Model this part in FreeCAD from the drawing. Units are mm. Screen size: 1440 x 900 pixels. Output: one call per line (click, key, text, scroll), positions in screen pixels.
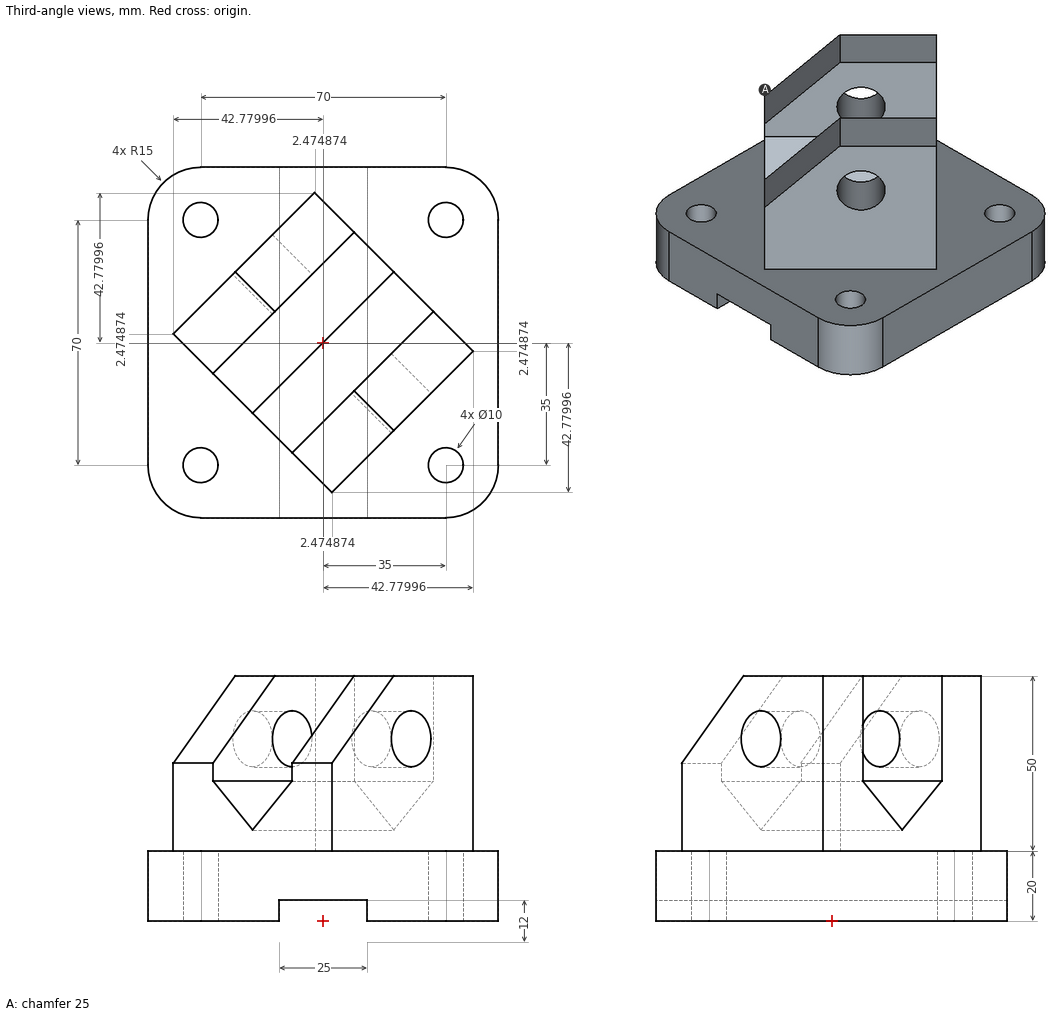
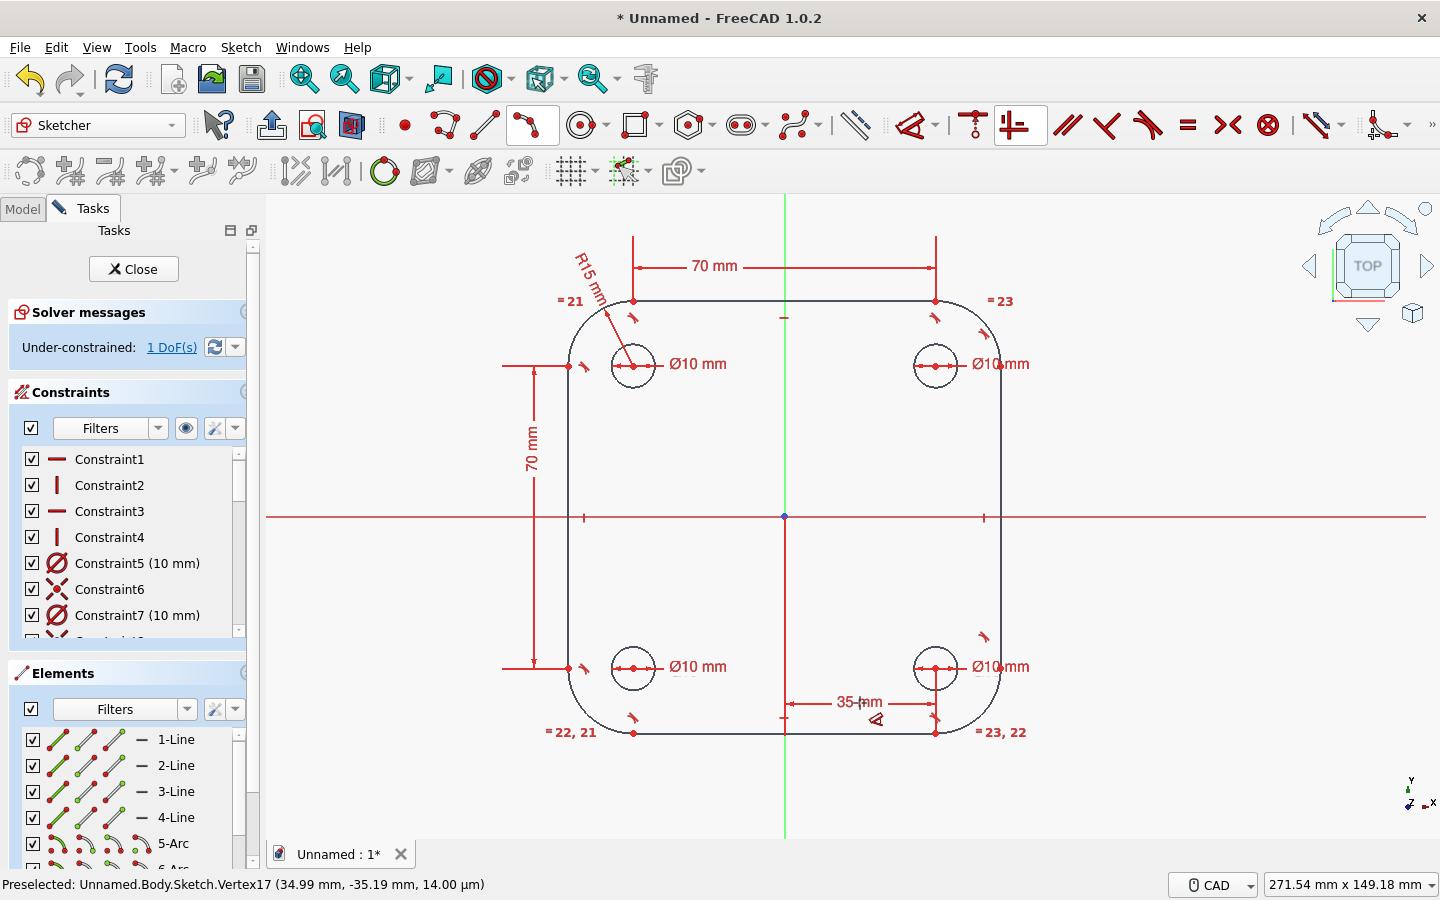
click(936, 669)
click(970, 593)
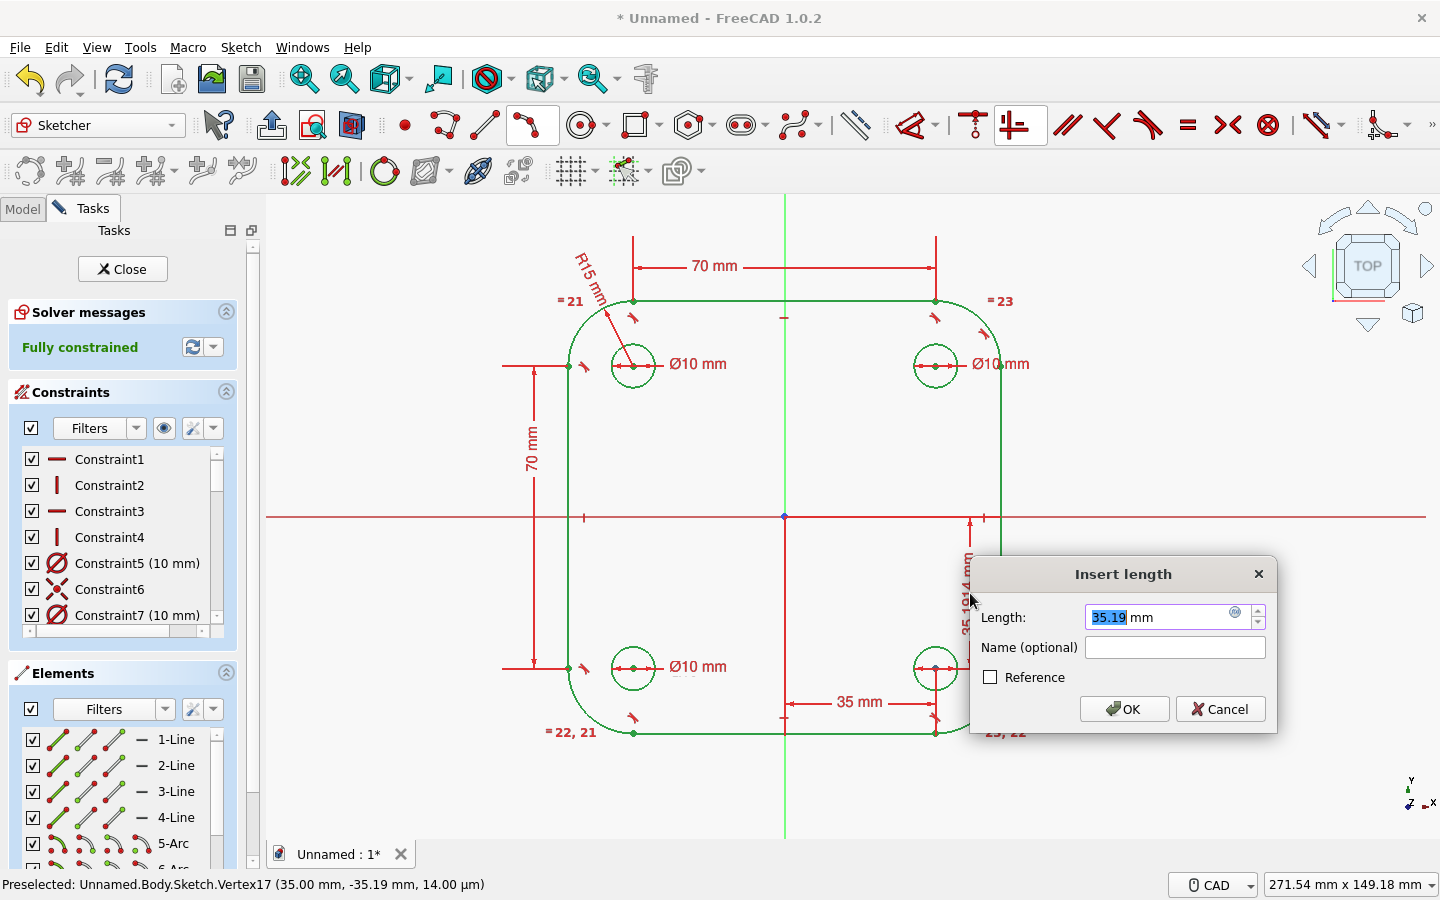
text(35)
key(Return)
key(Escape)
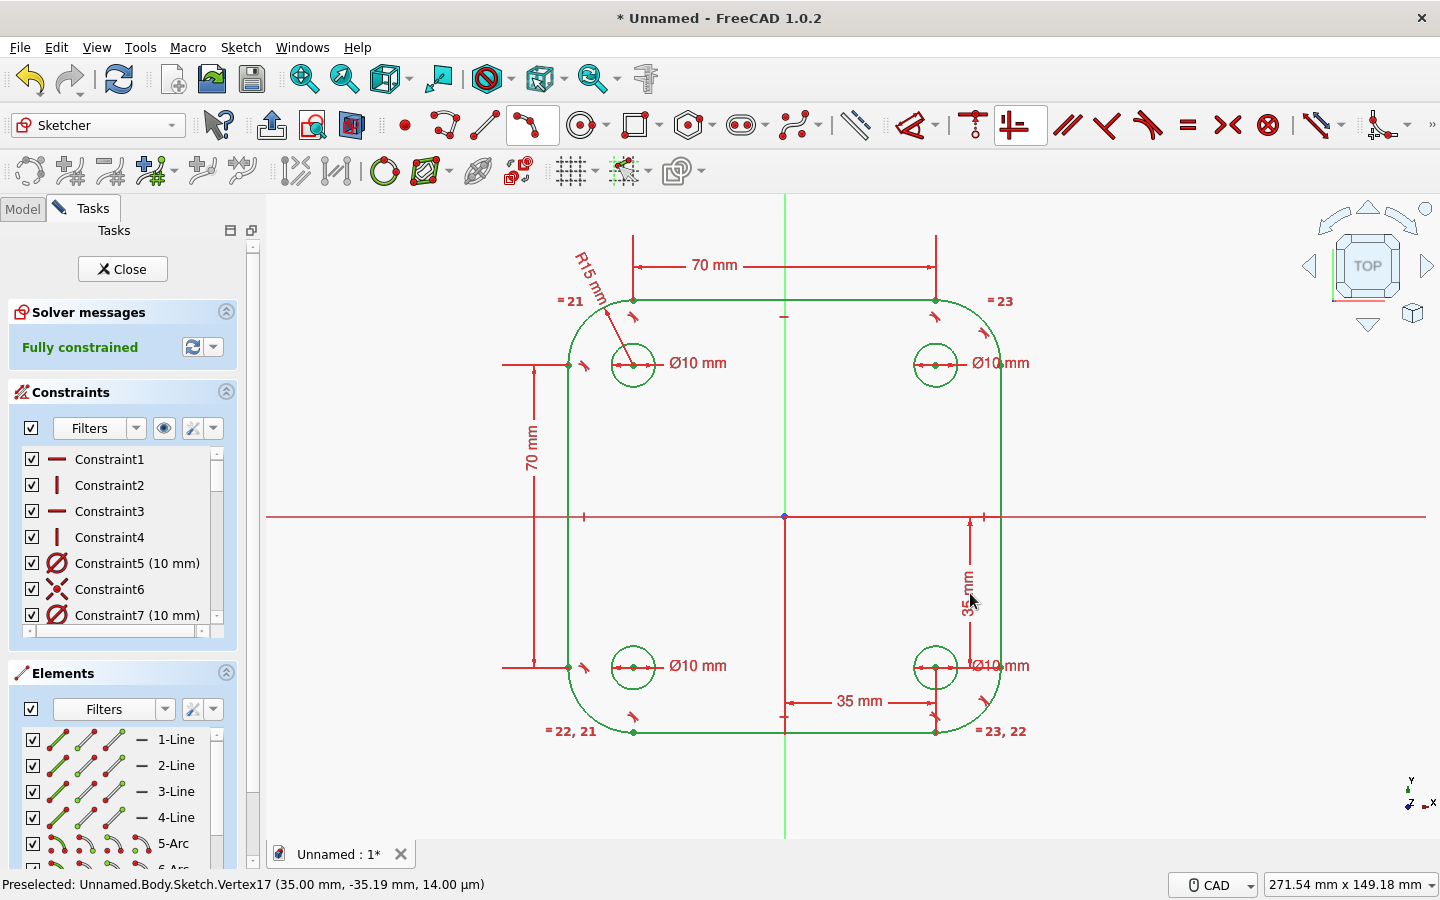
click(123, 269)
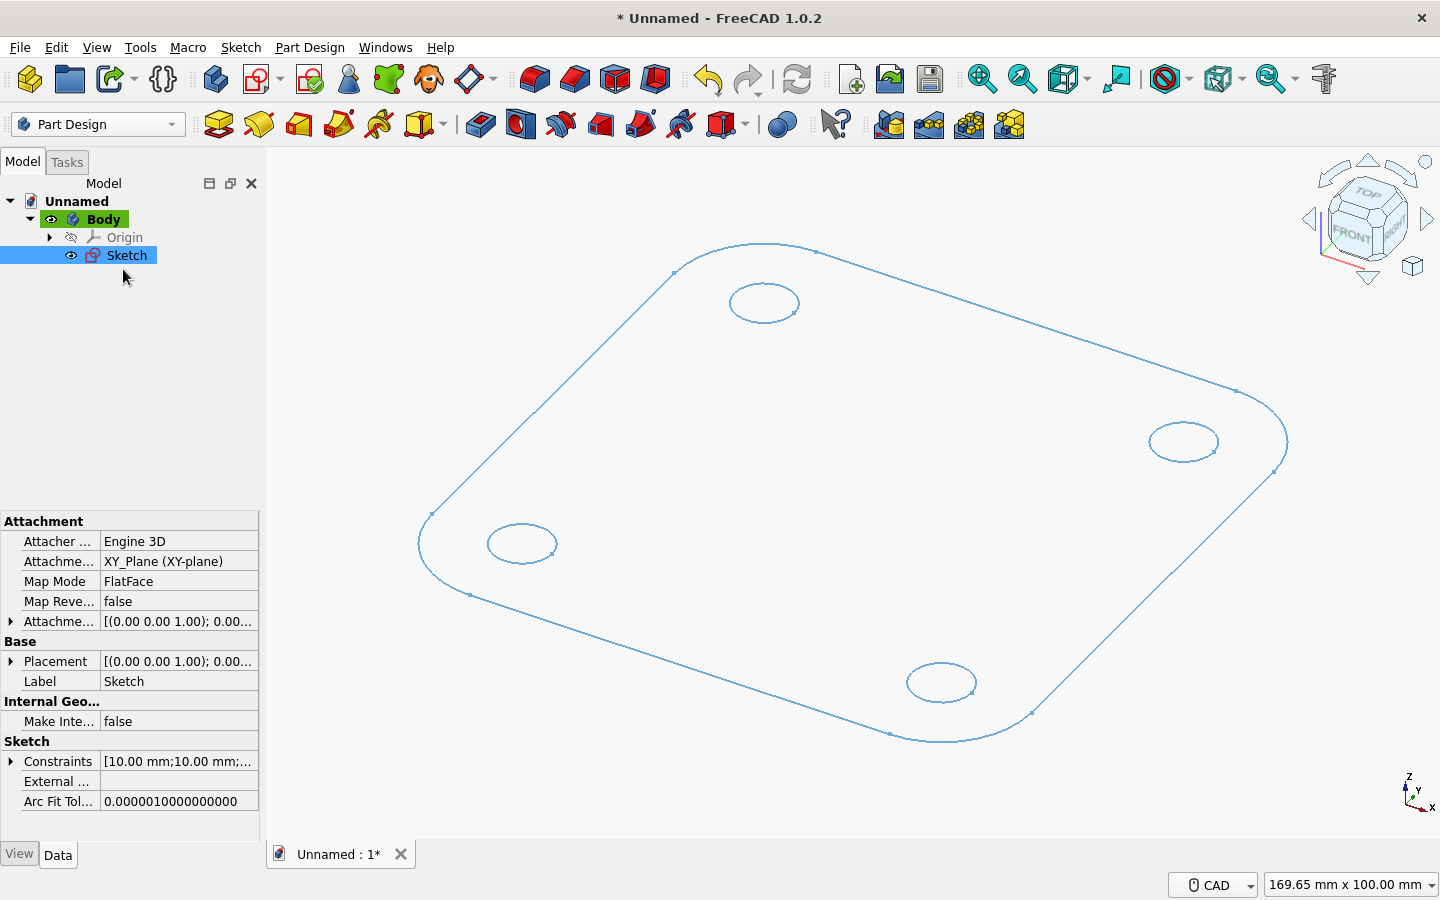
click(220, 124)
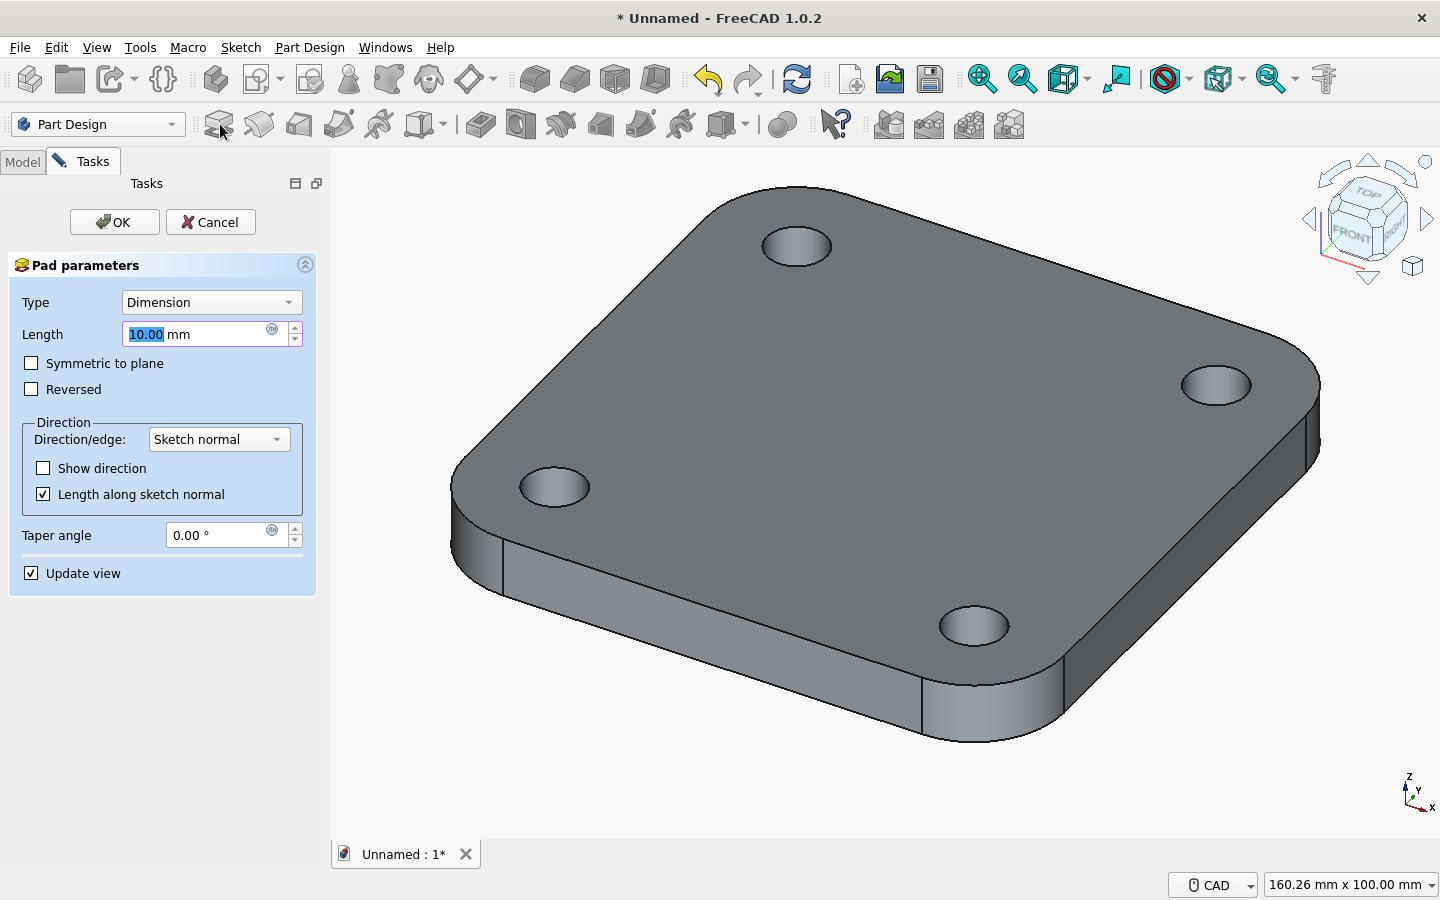
text(20)
key(Tab)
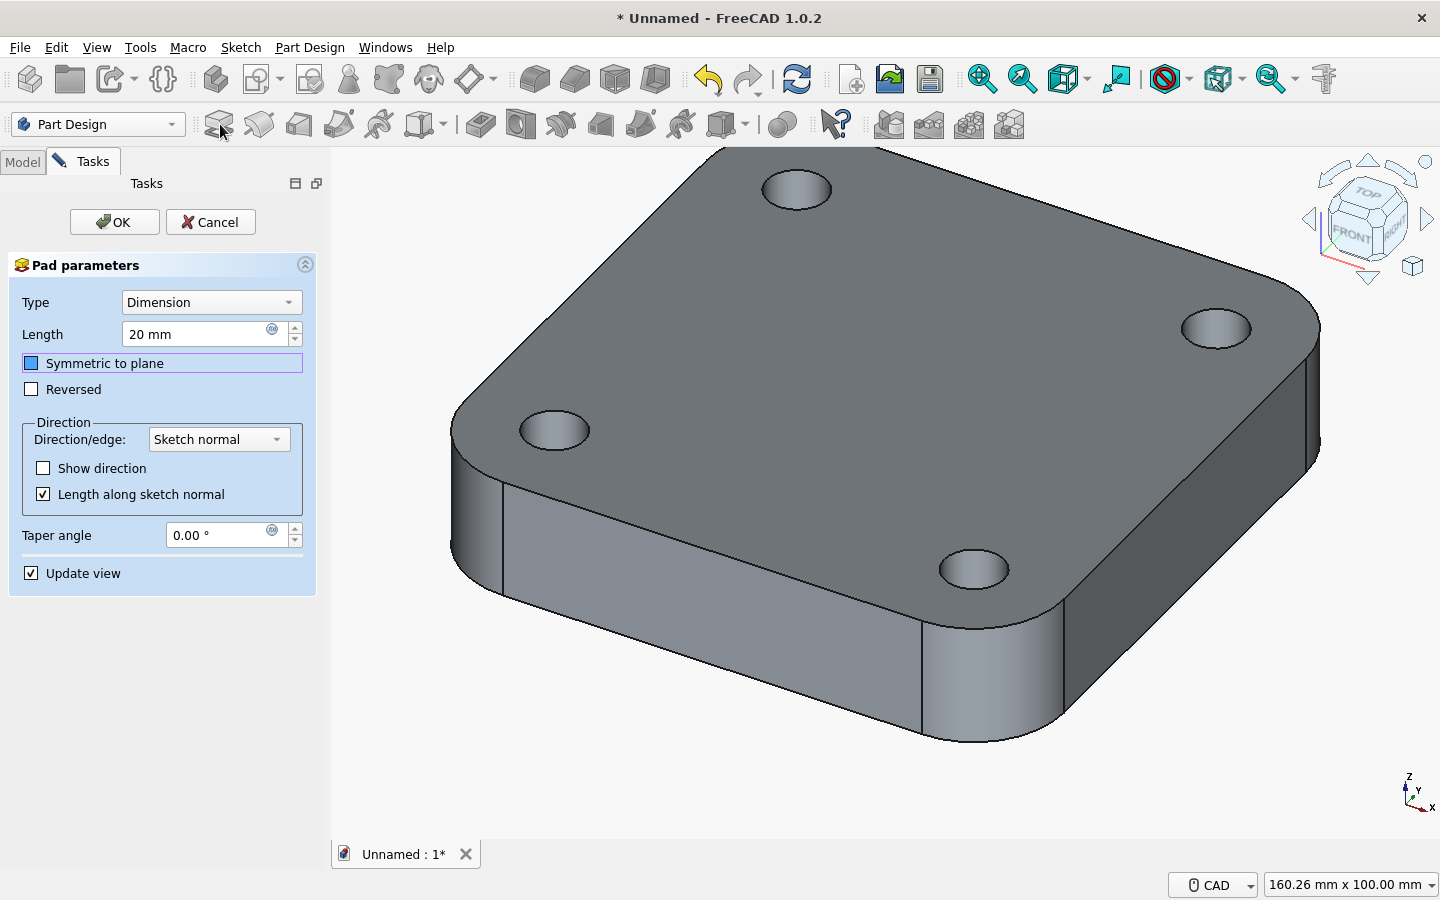
click(115, 222)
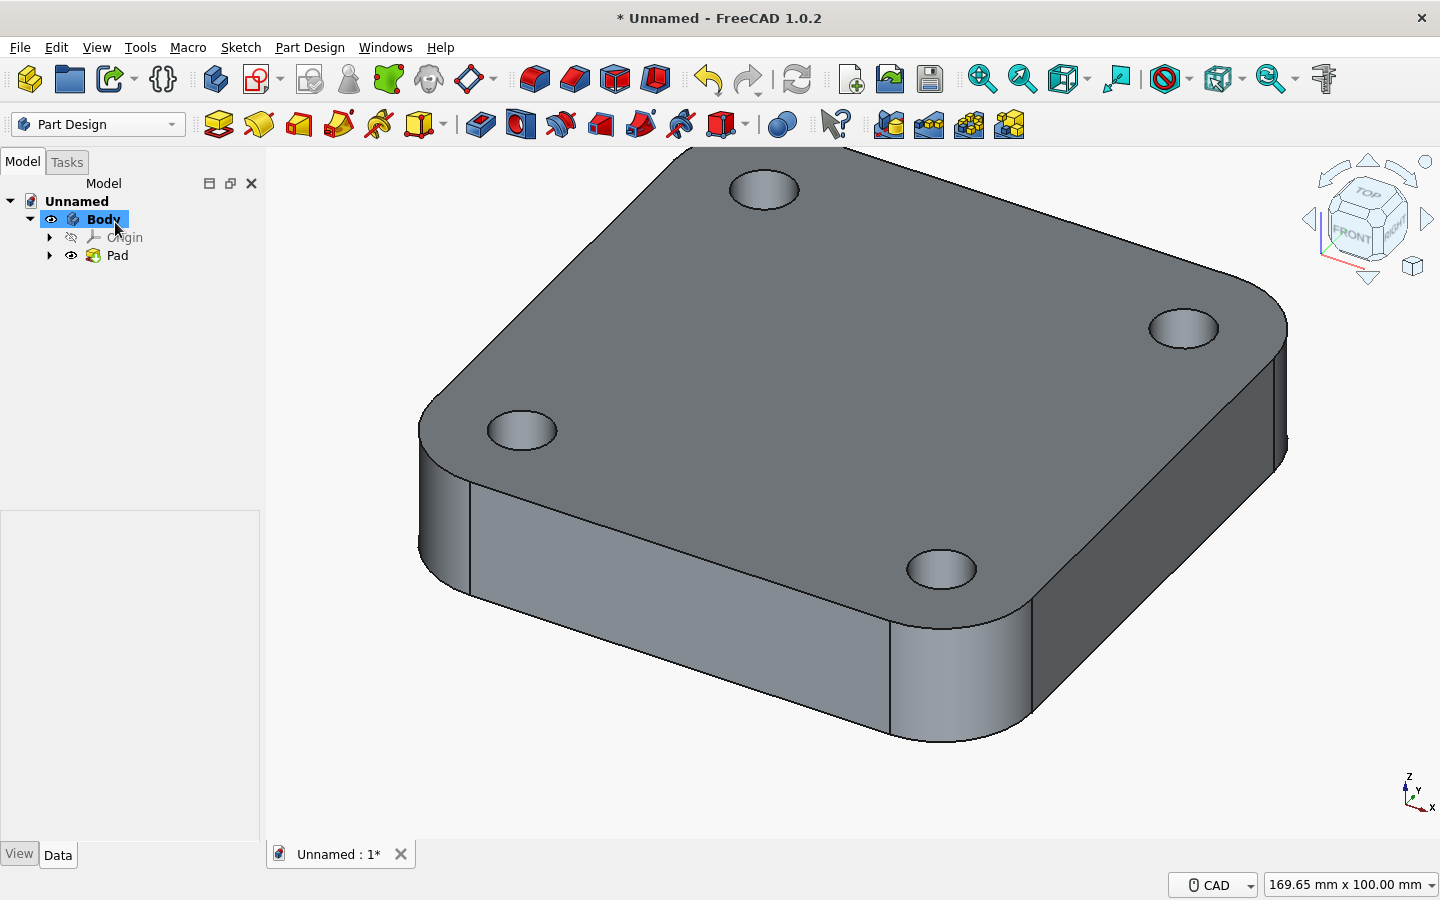
click(984, 80)